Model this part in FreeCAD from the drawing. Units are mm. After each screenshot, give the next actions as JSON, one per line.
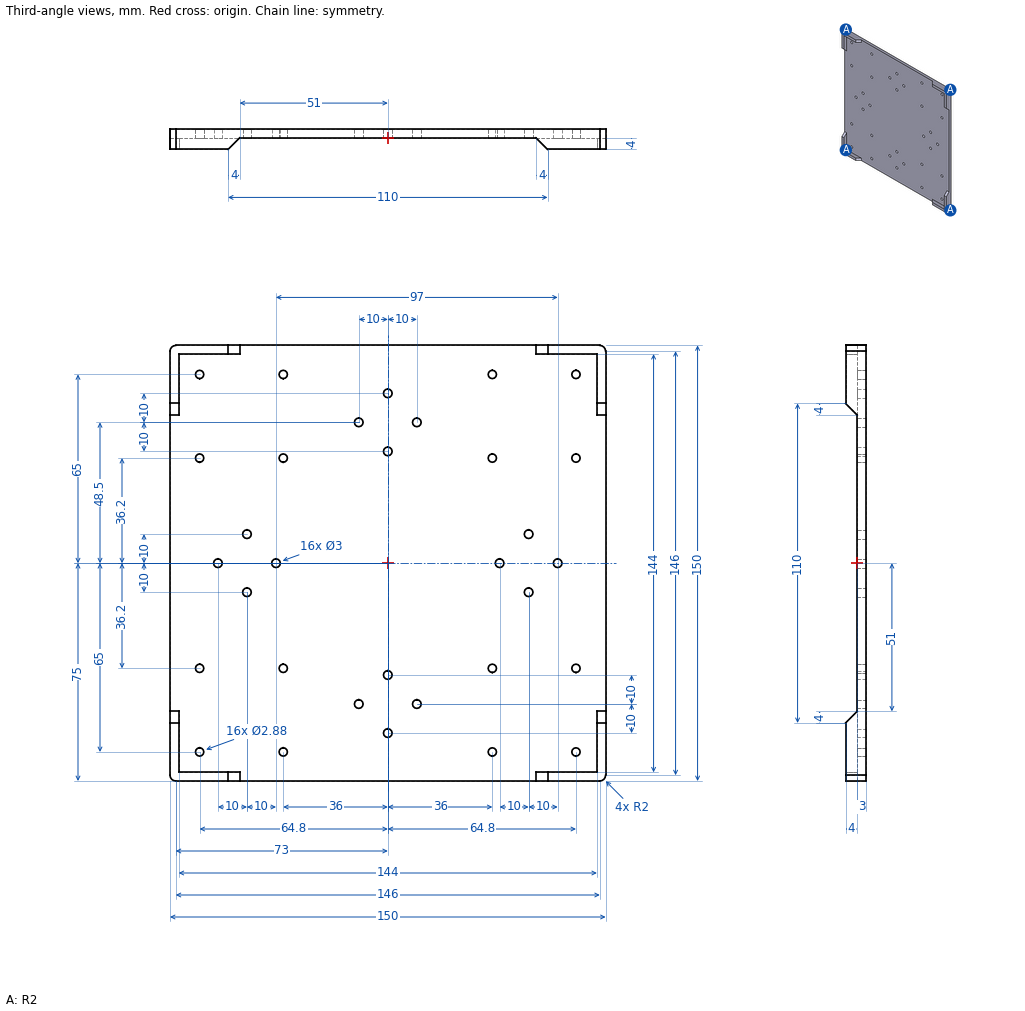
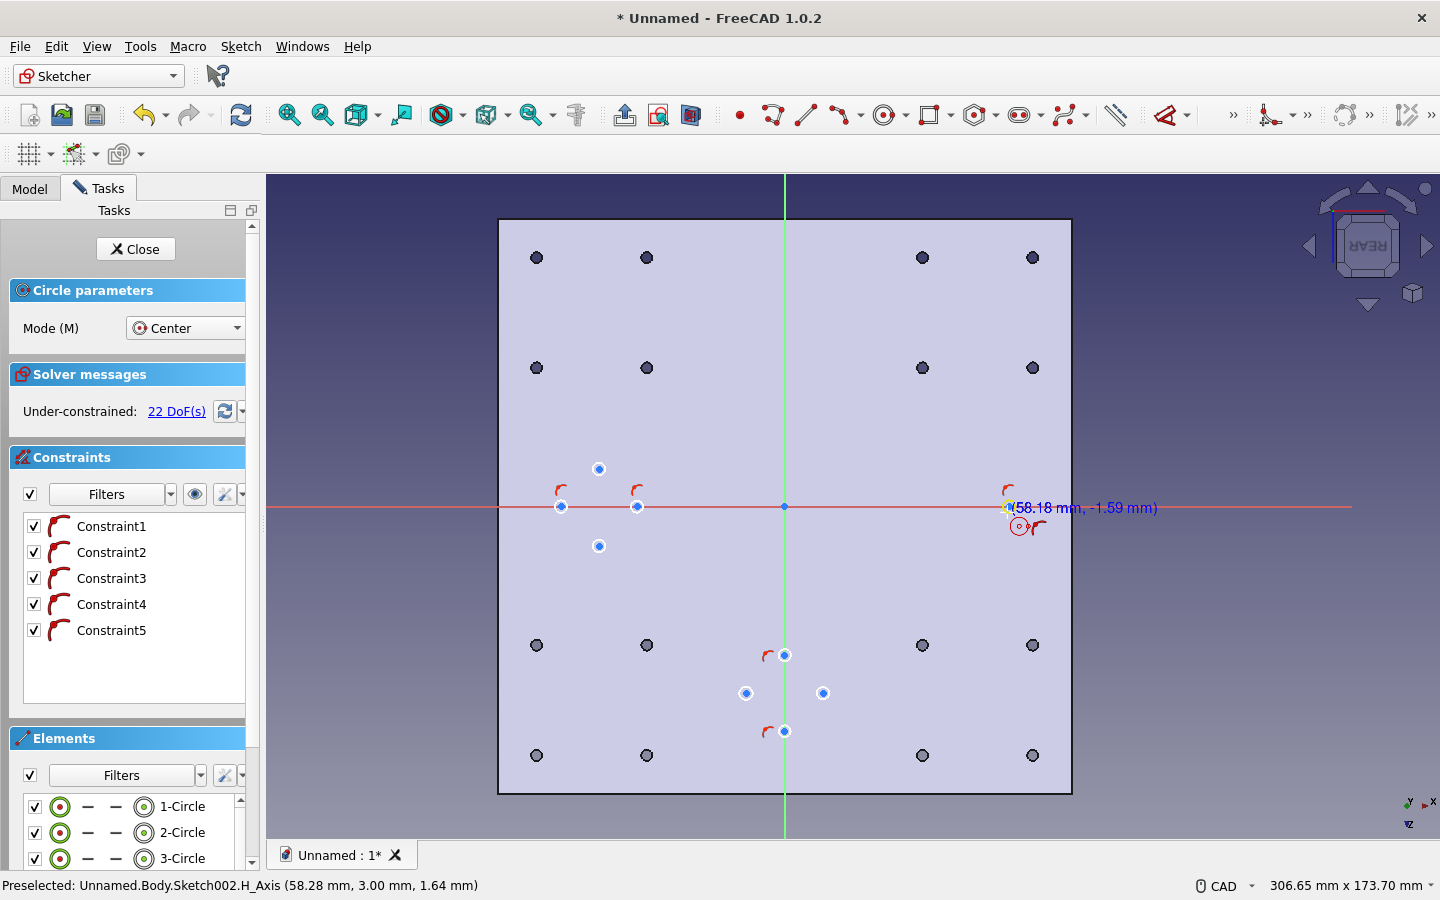
{"action": "left_click", "coordinate": [970, 468]}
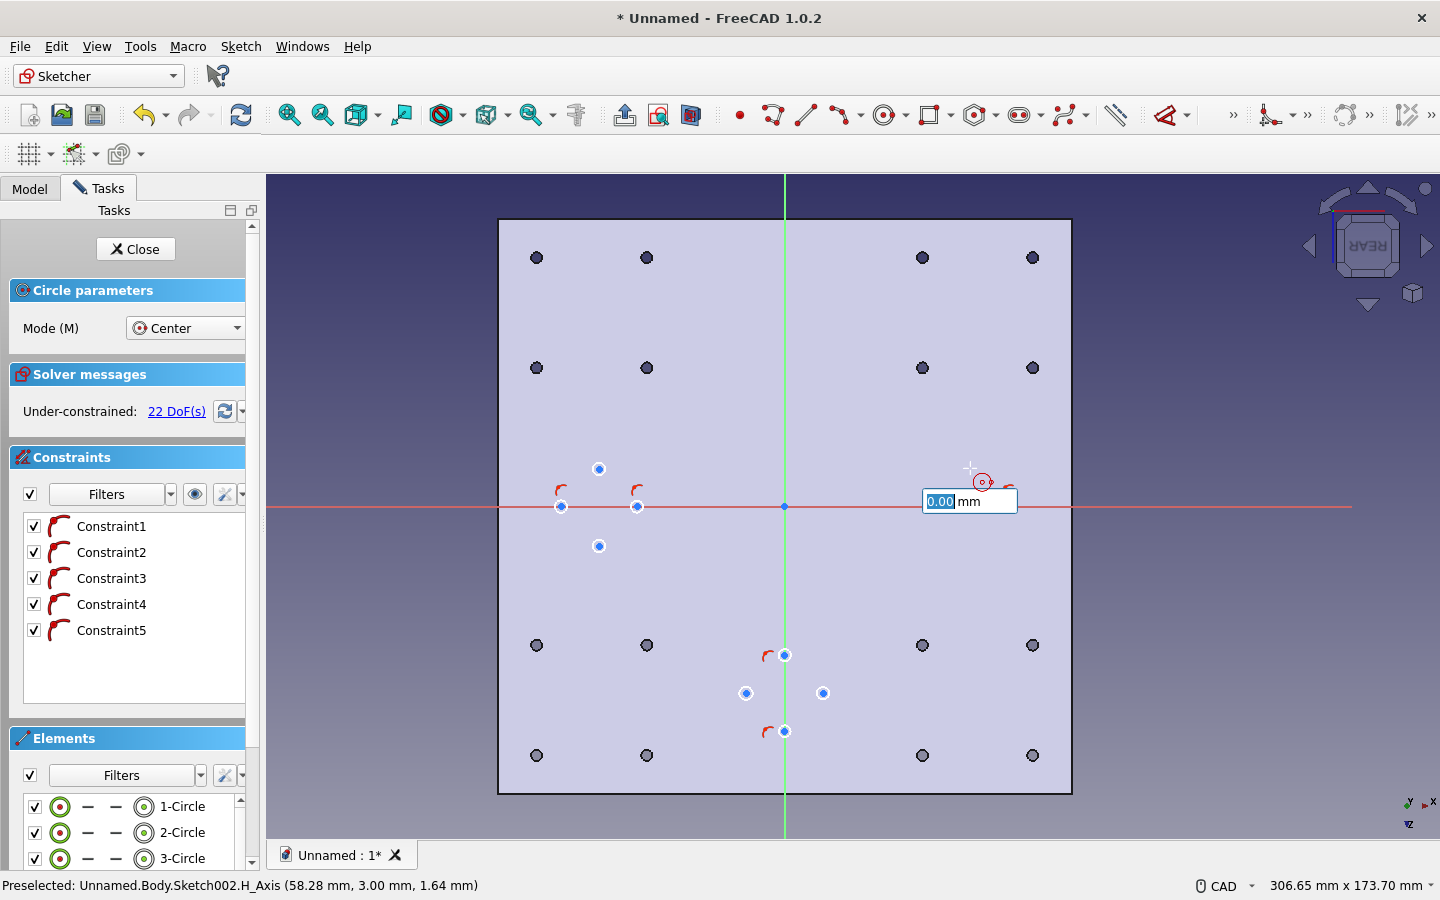
{"action": "scroll", "coordinate": [974, 464], "scroll_direction": "up", "scroll_amount": 6}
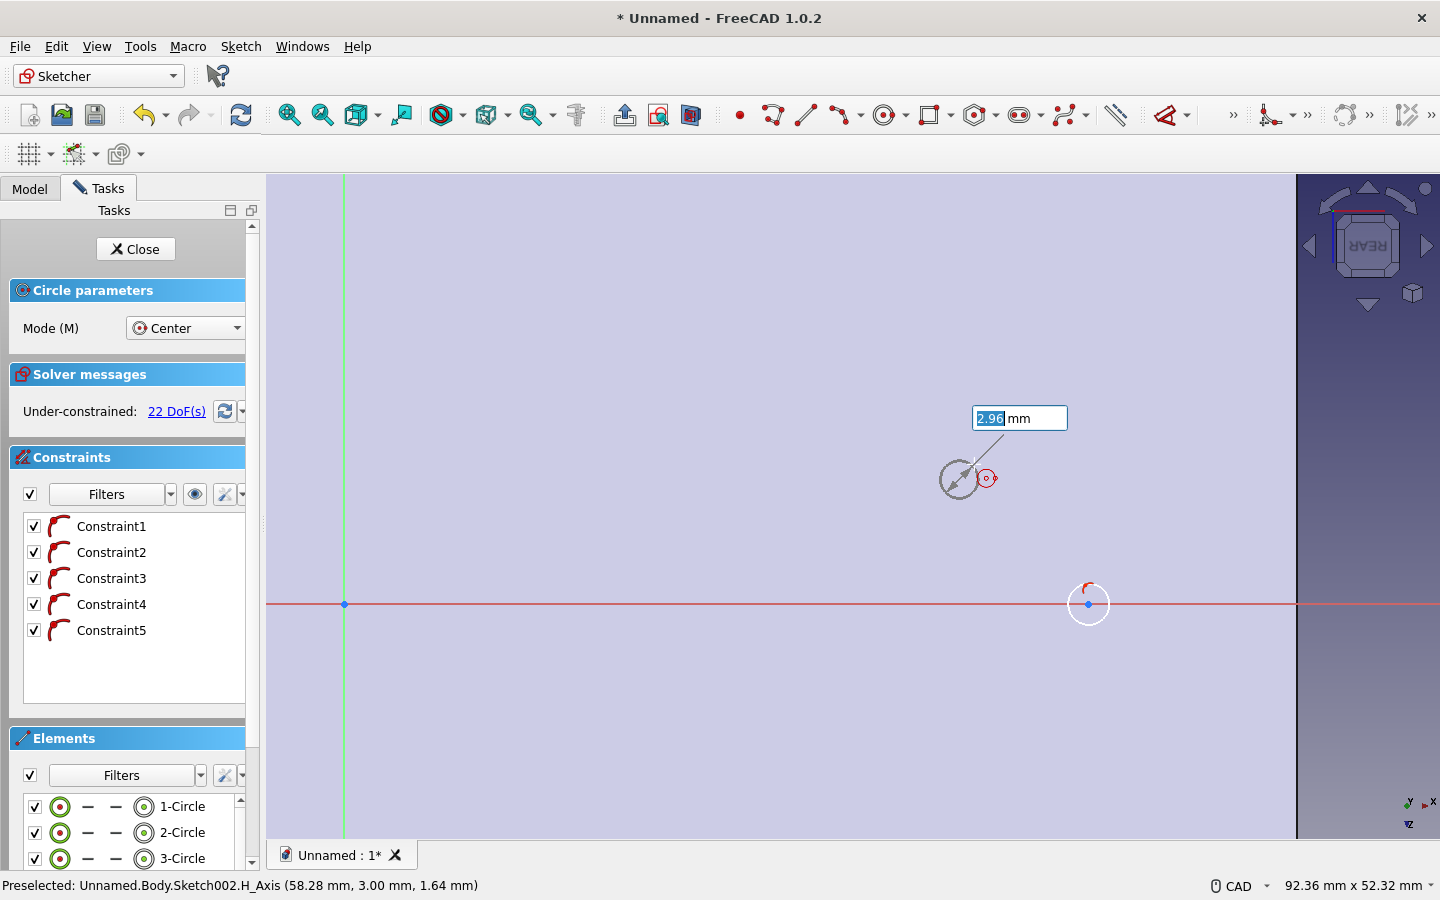
{"action": "left_click", "coordinate": [974, 464]}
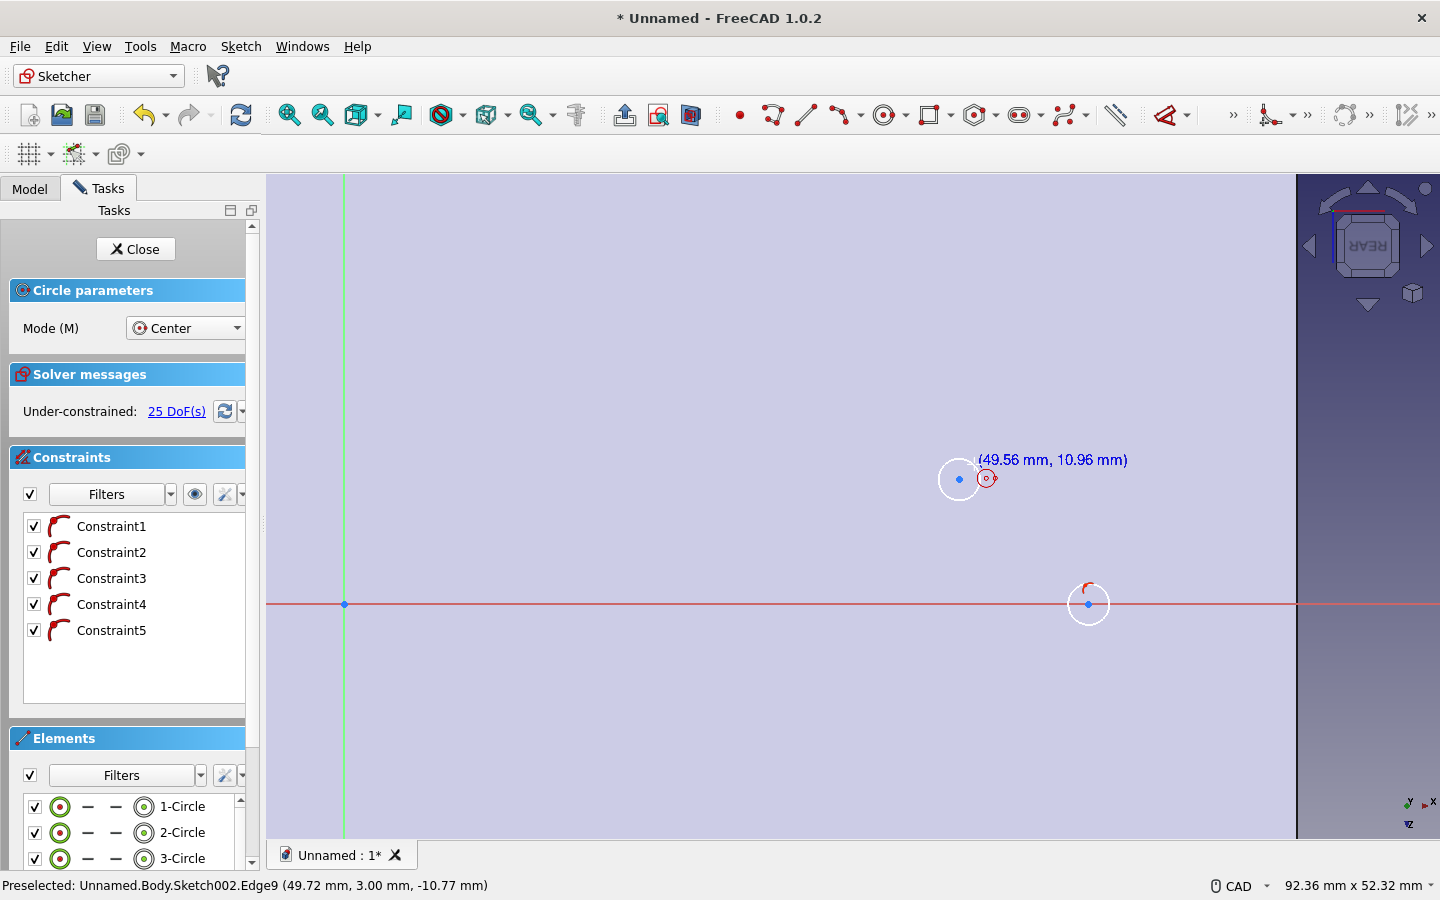
{"action": "scroll", "coordinate": [974, 464], "scroll_direction": "down", "scroll_amount": 6}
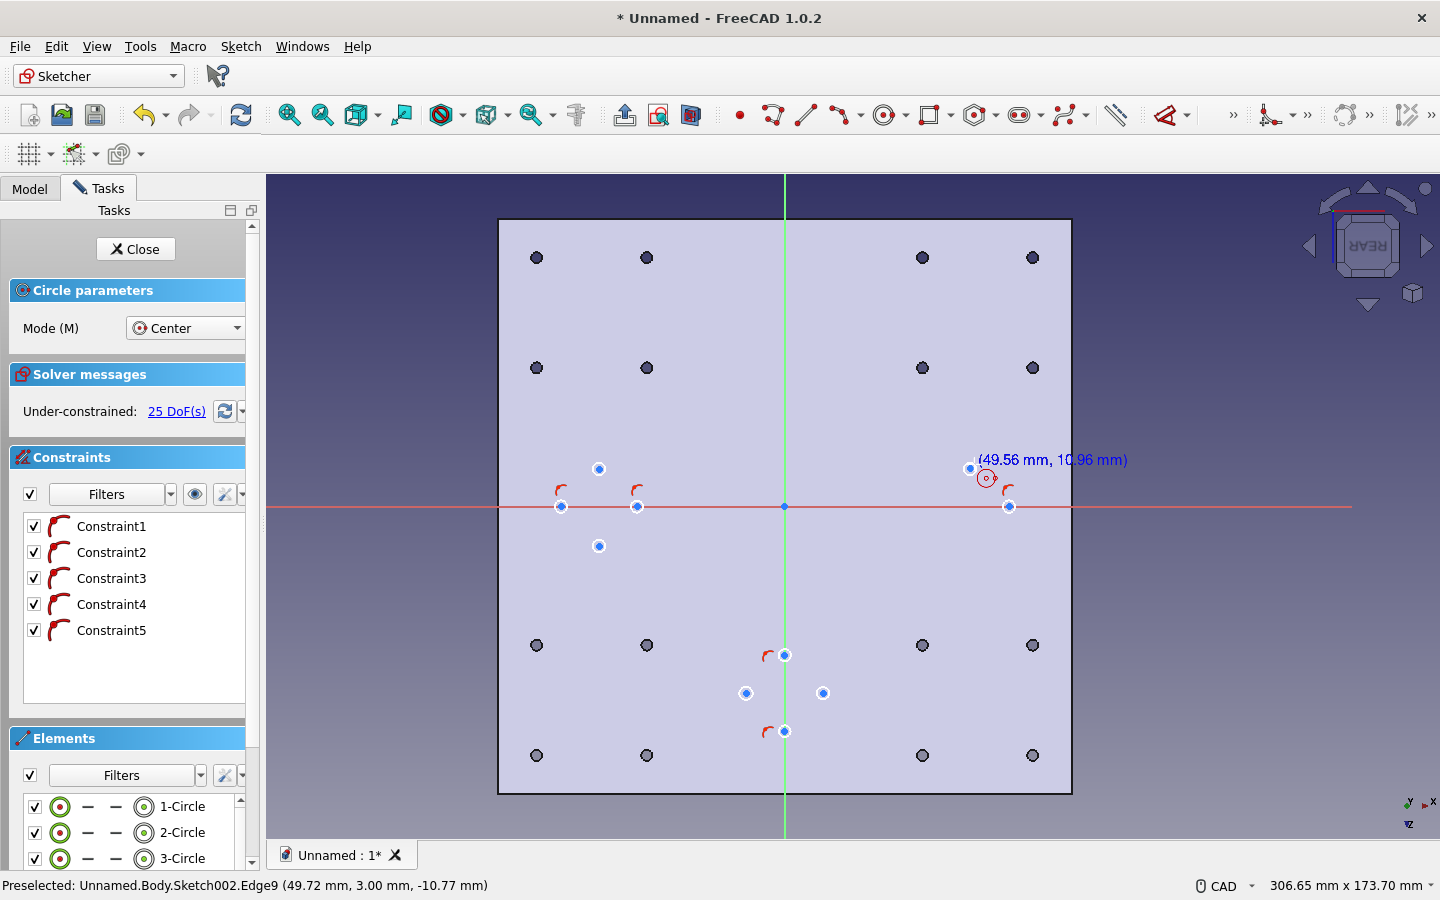
{"action": "left_click", "coordinate": [932, 507]}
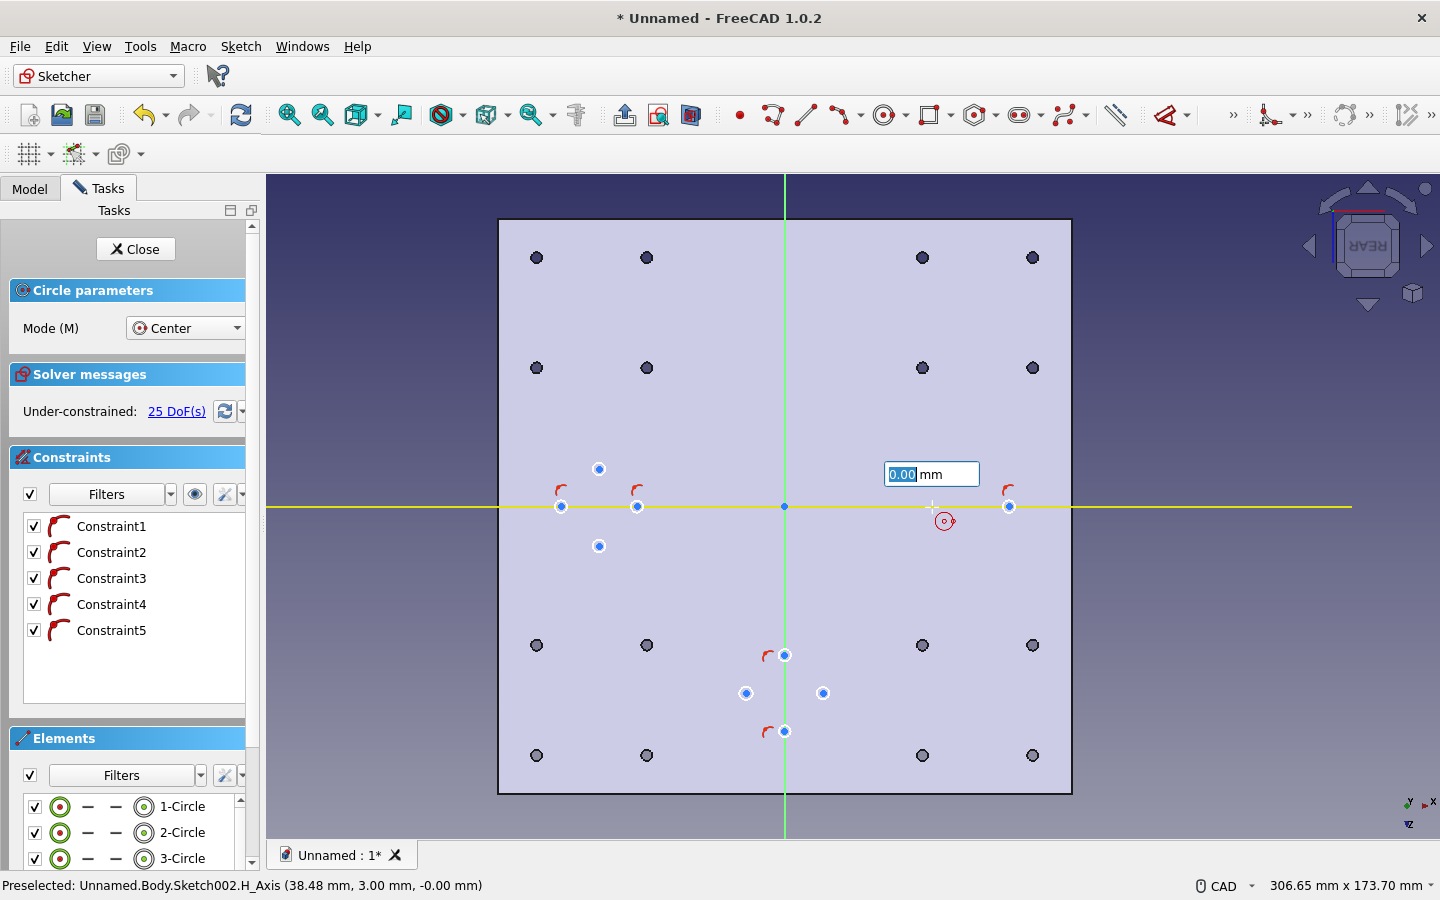
{"action": "scroll", "coordinate": [930, 512], "scroll_direction": "up", "scroll_amount": 6}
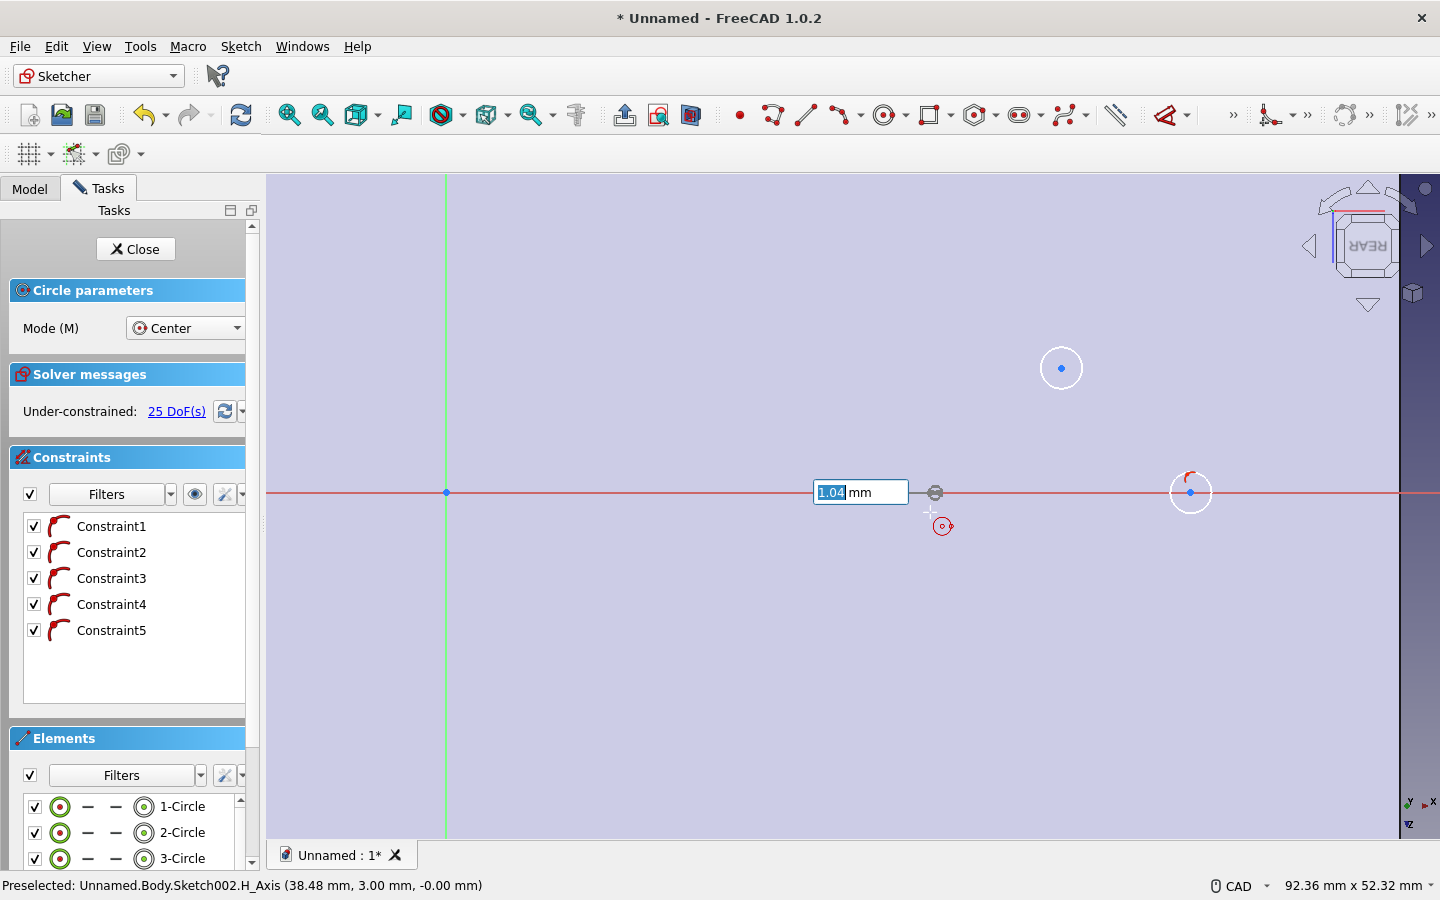
{"action": "left_click", "coordinate": [929, 511]}